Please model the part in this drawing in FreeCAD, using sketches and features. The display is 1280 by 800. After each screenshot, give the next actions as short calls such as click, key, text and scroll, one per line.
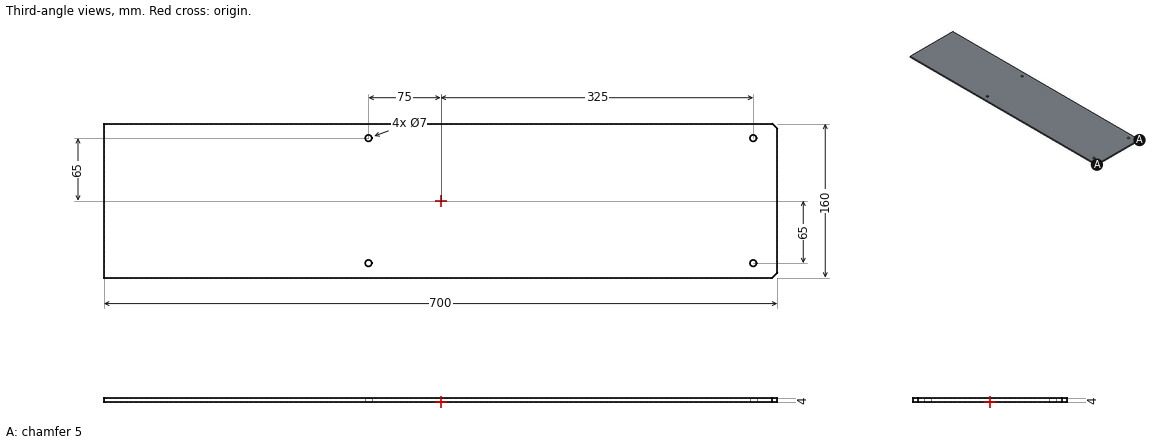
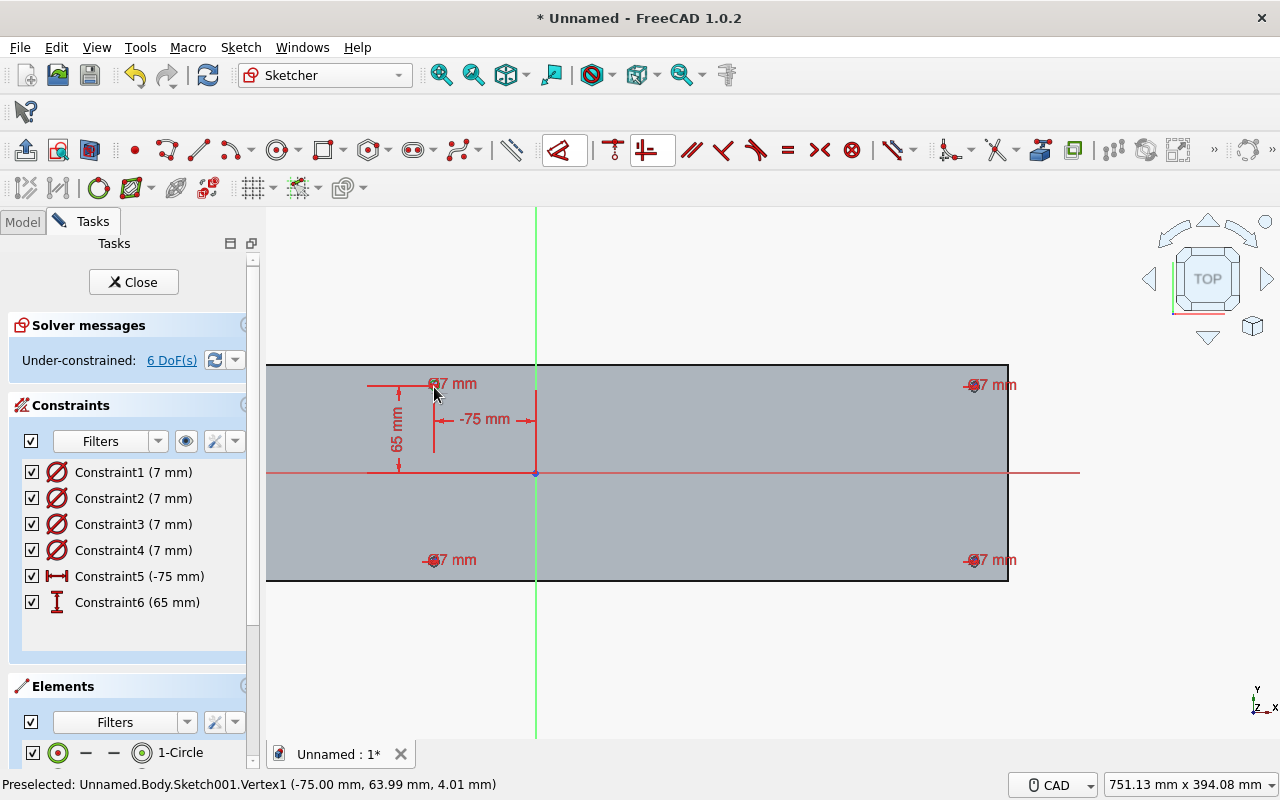
click(974, 387)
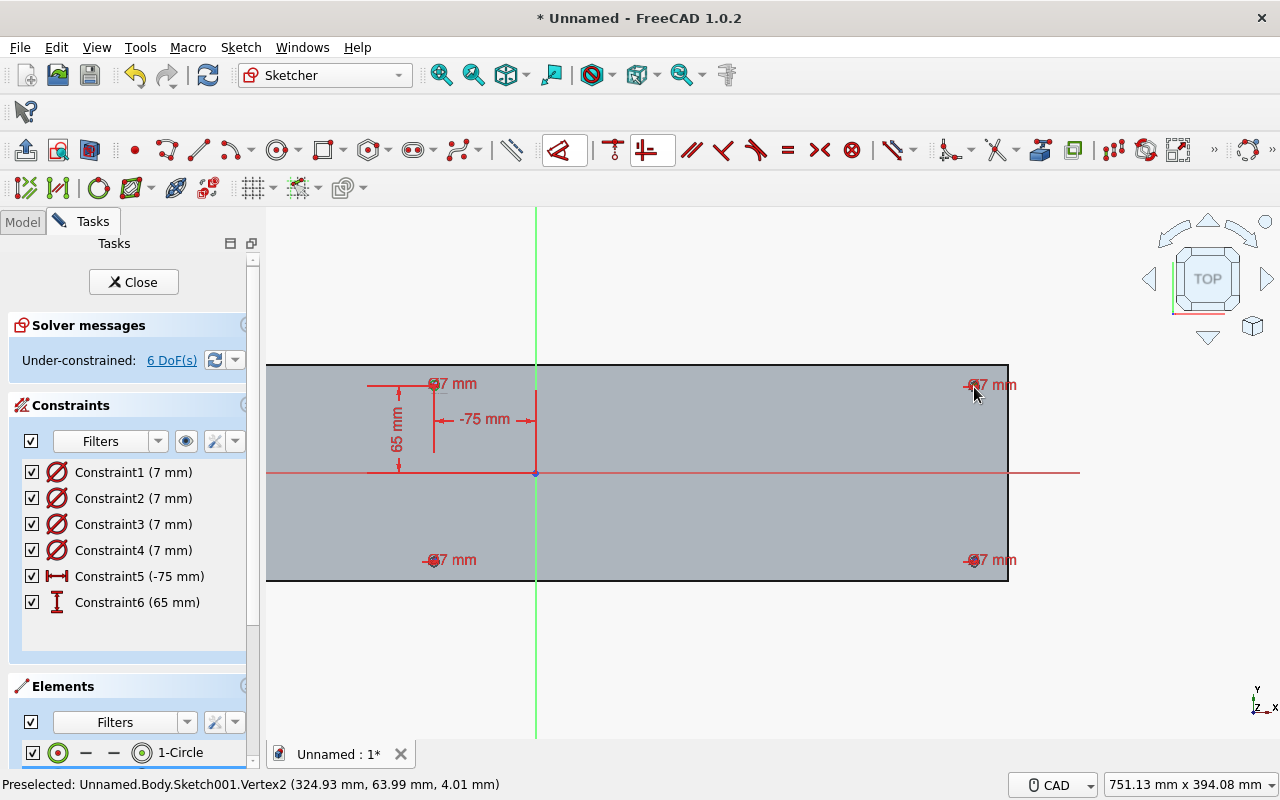
click(582, 150)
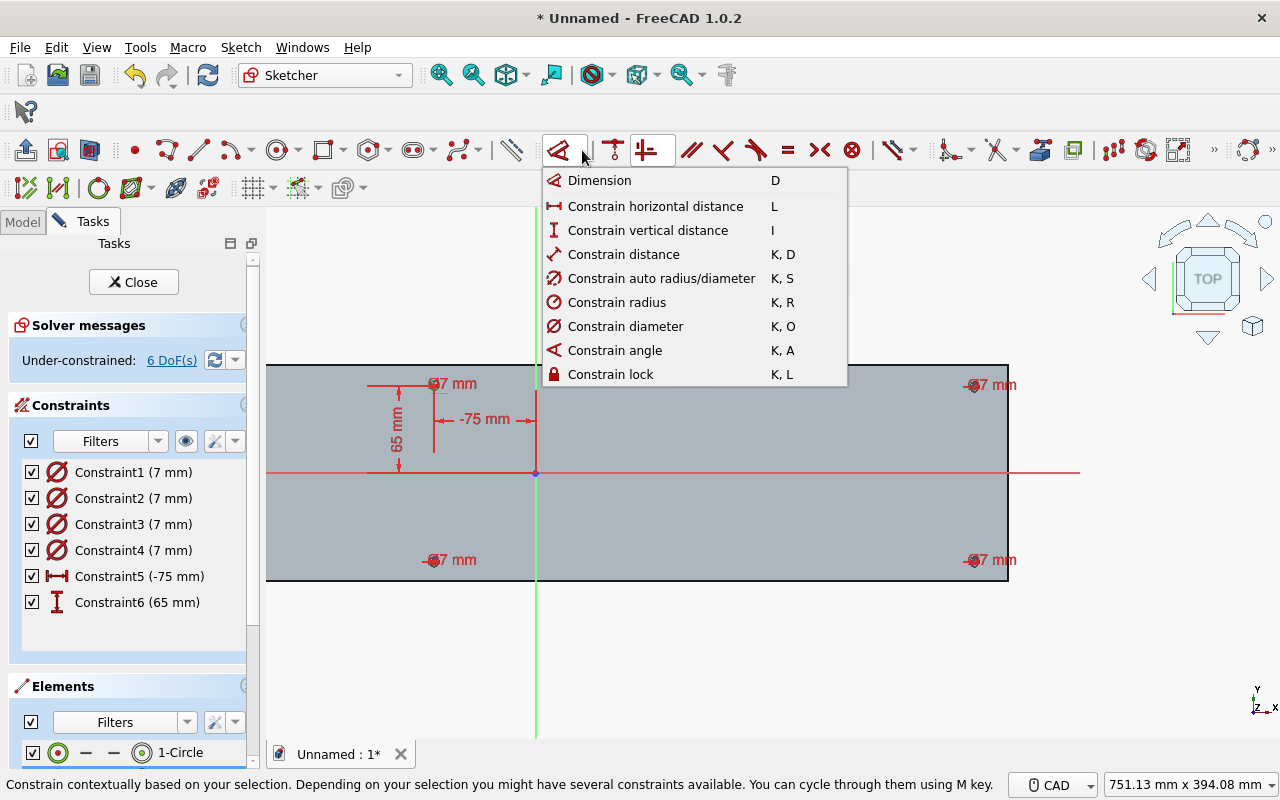
click(695, 230)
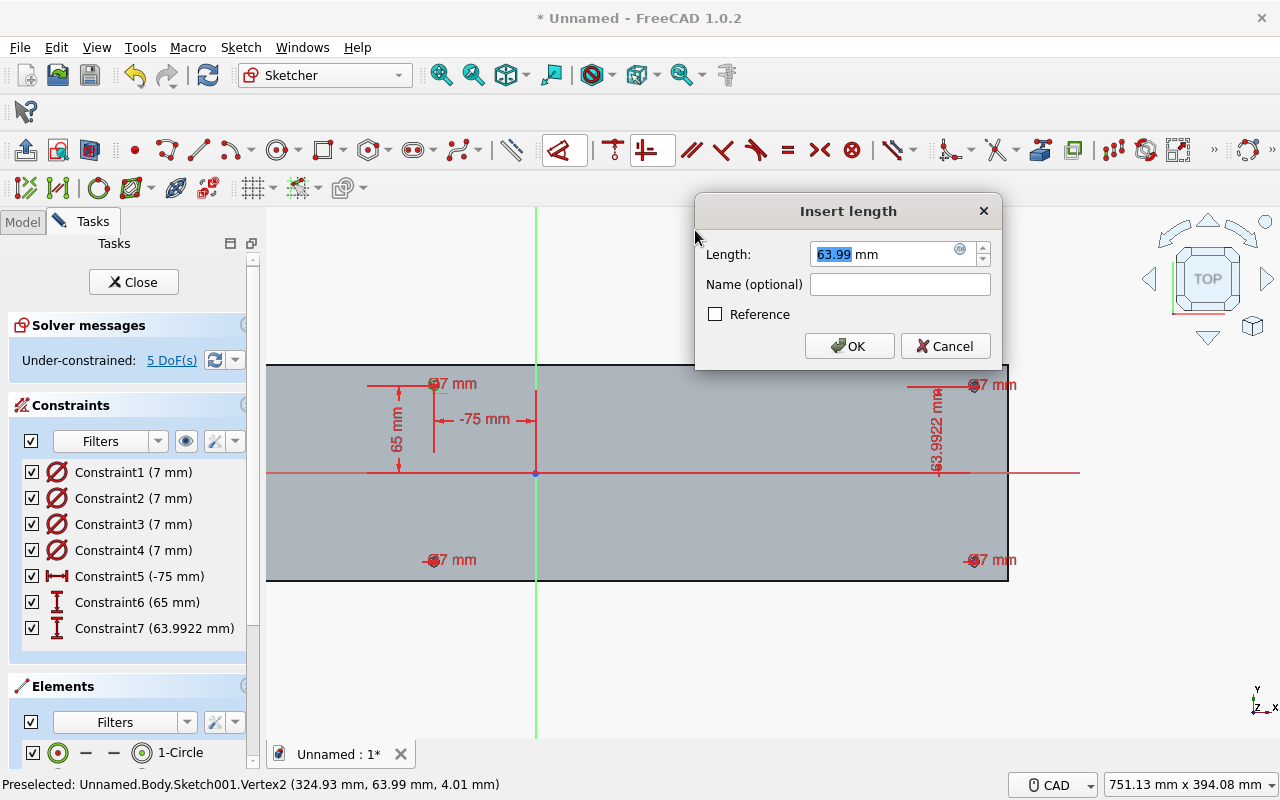
text(65)
key(Return)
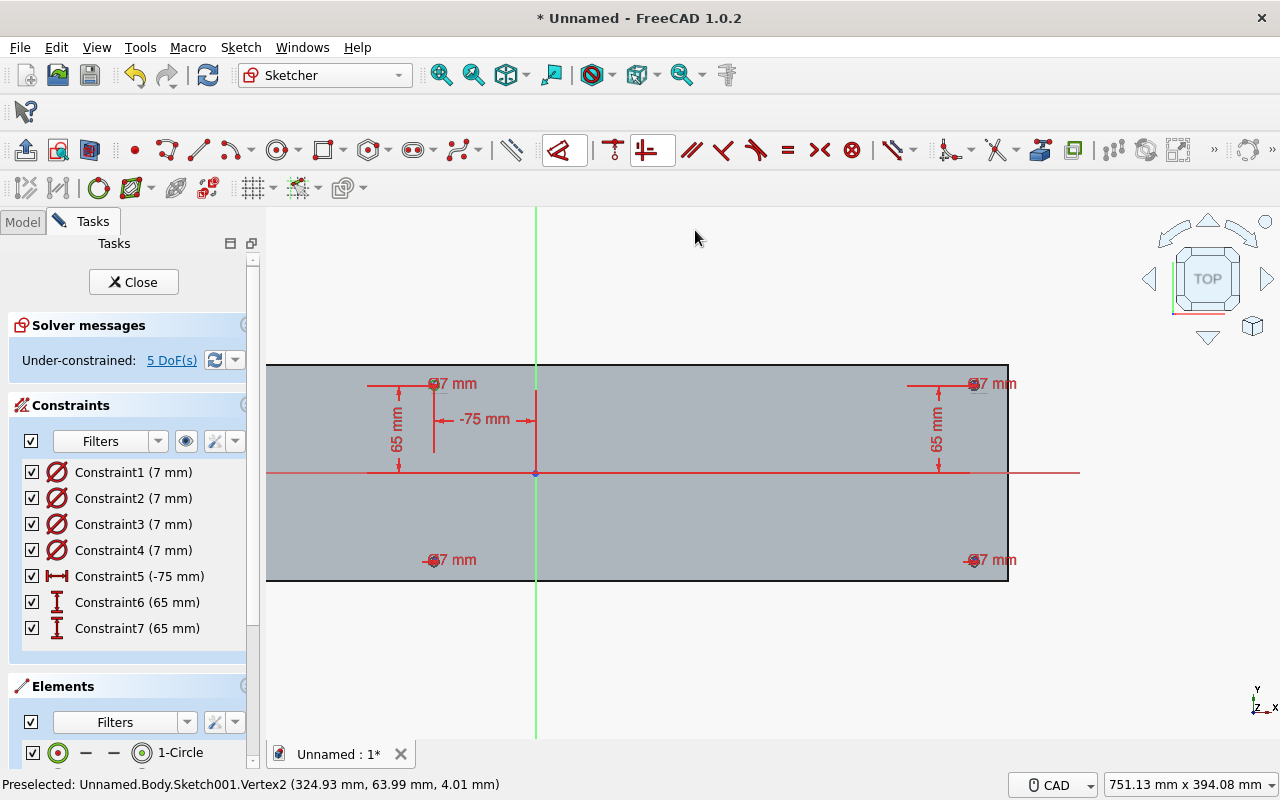
click(974, 562)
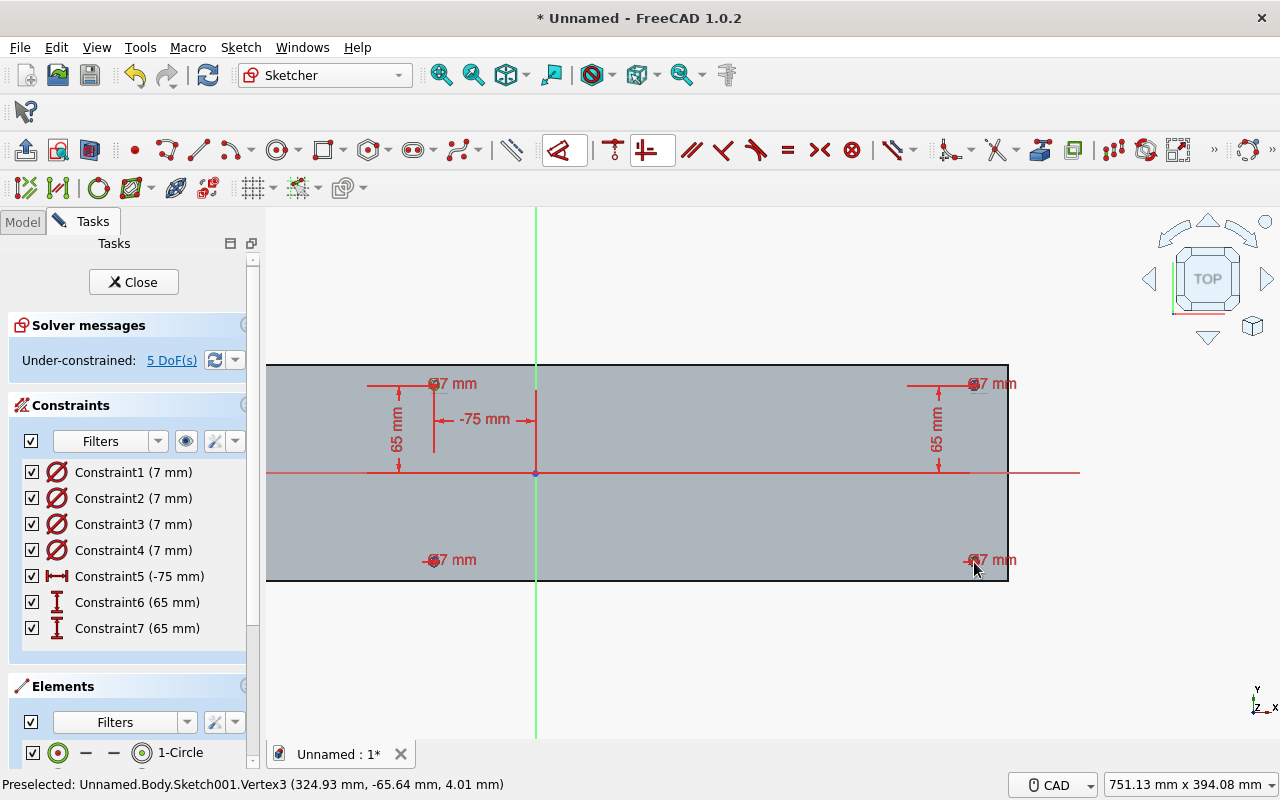
click(582, 150)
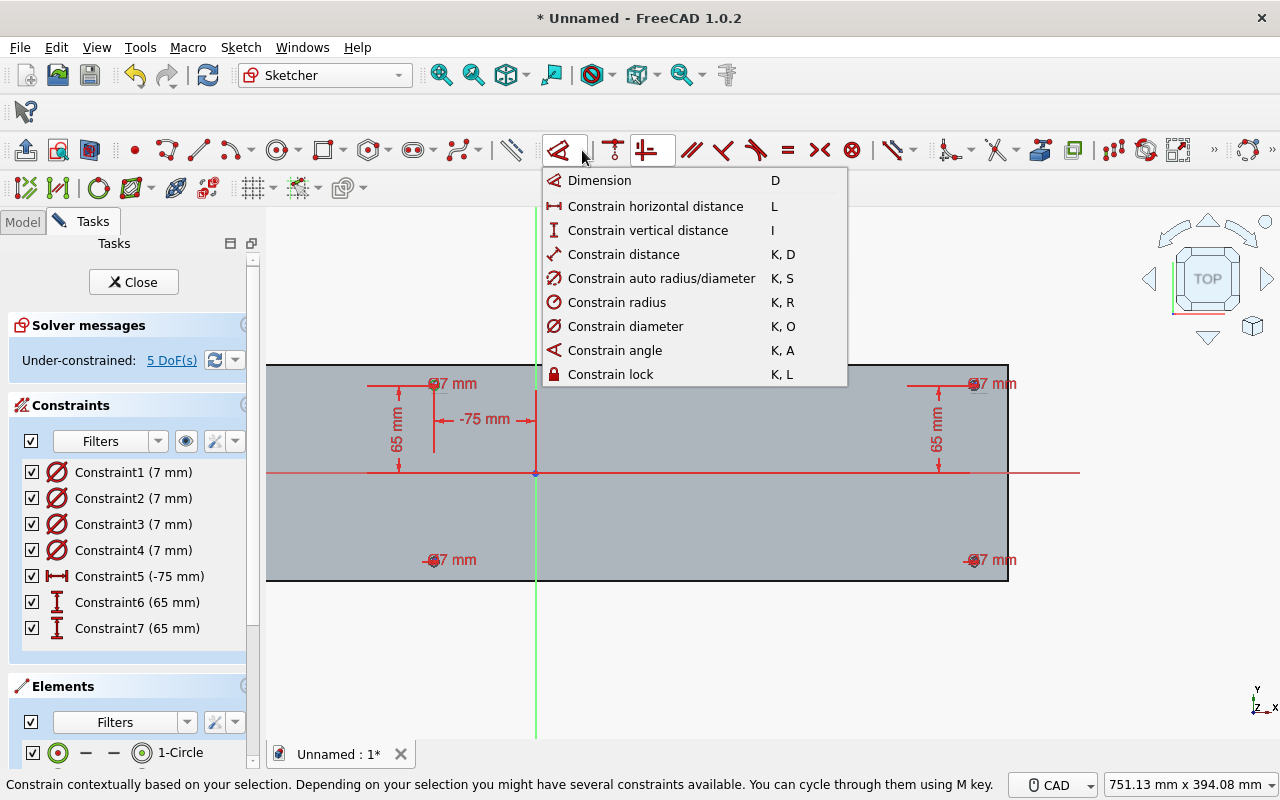
click(695, 230)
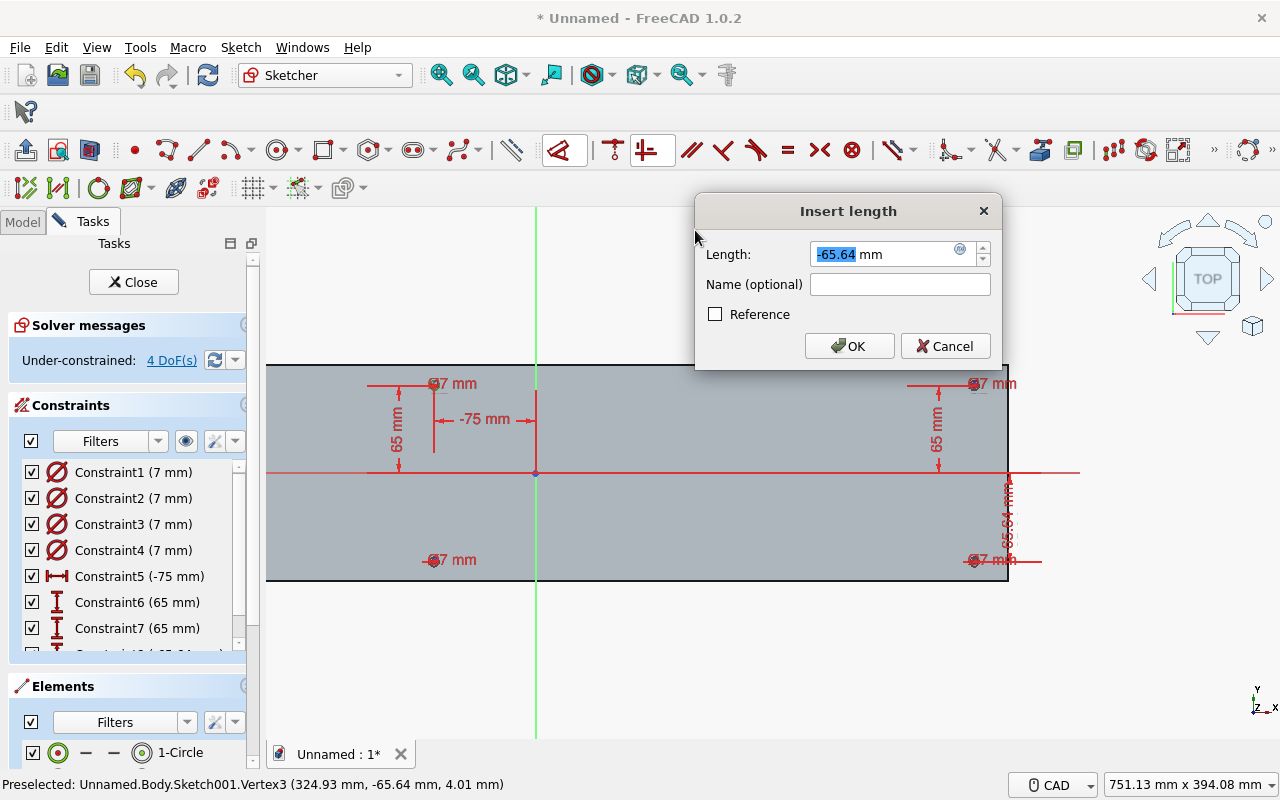
text(-65)
key(Return)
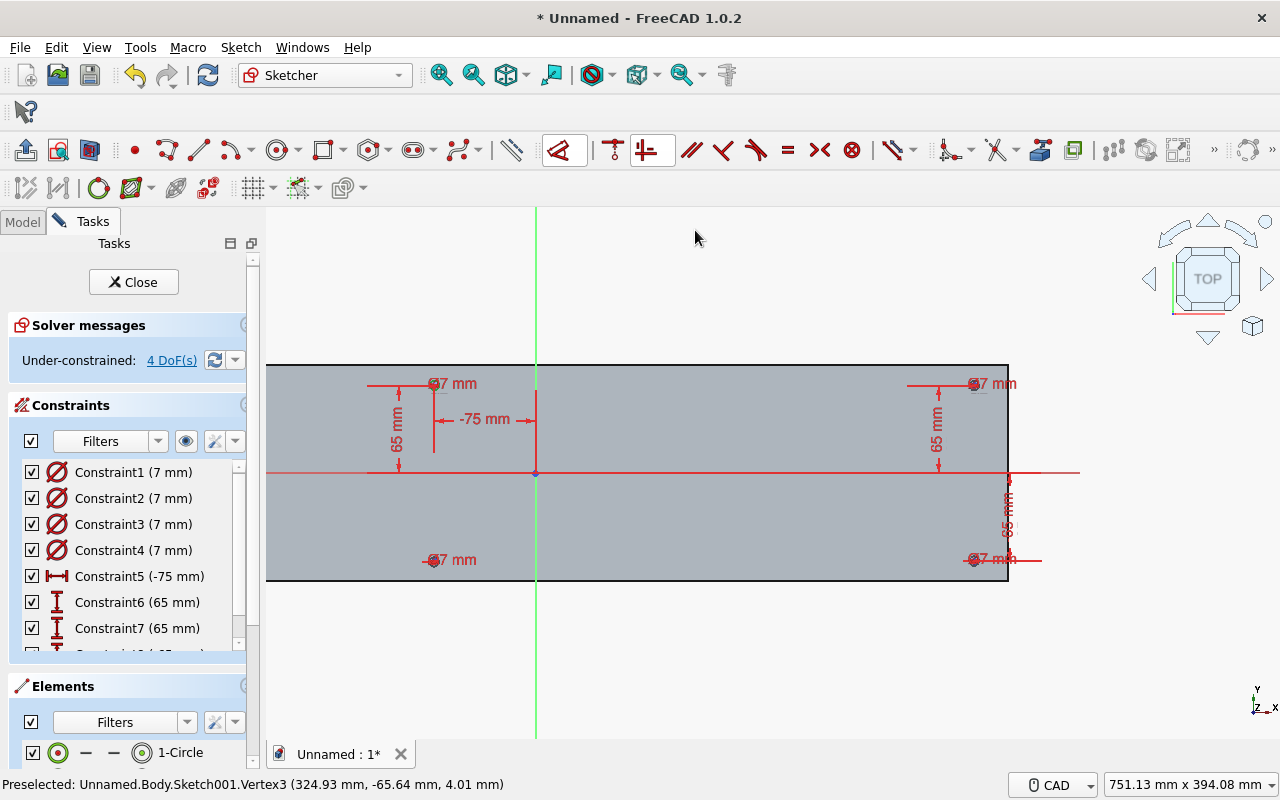
click(434, 562)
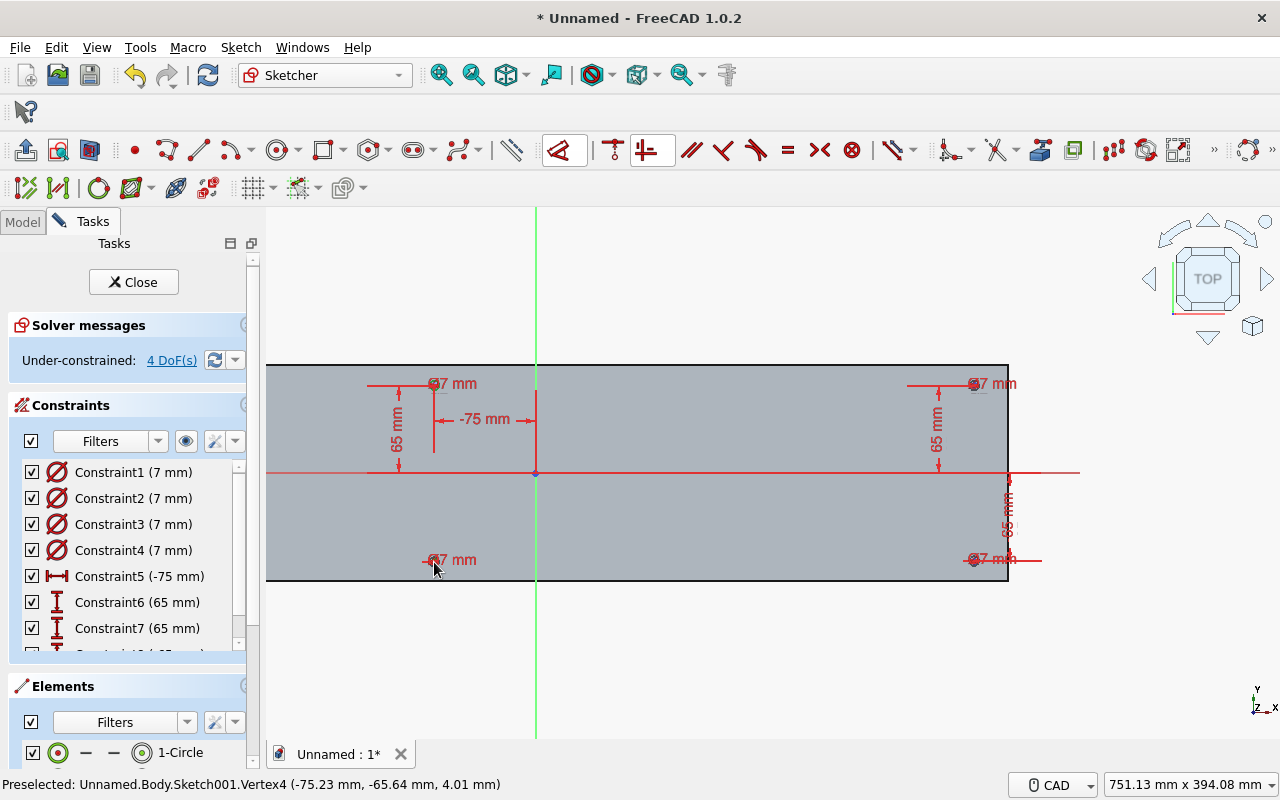
click(582, 150)